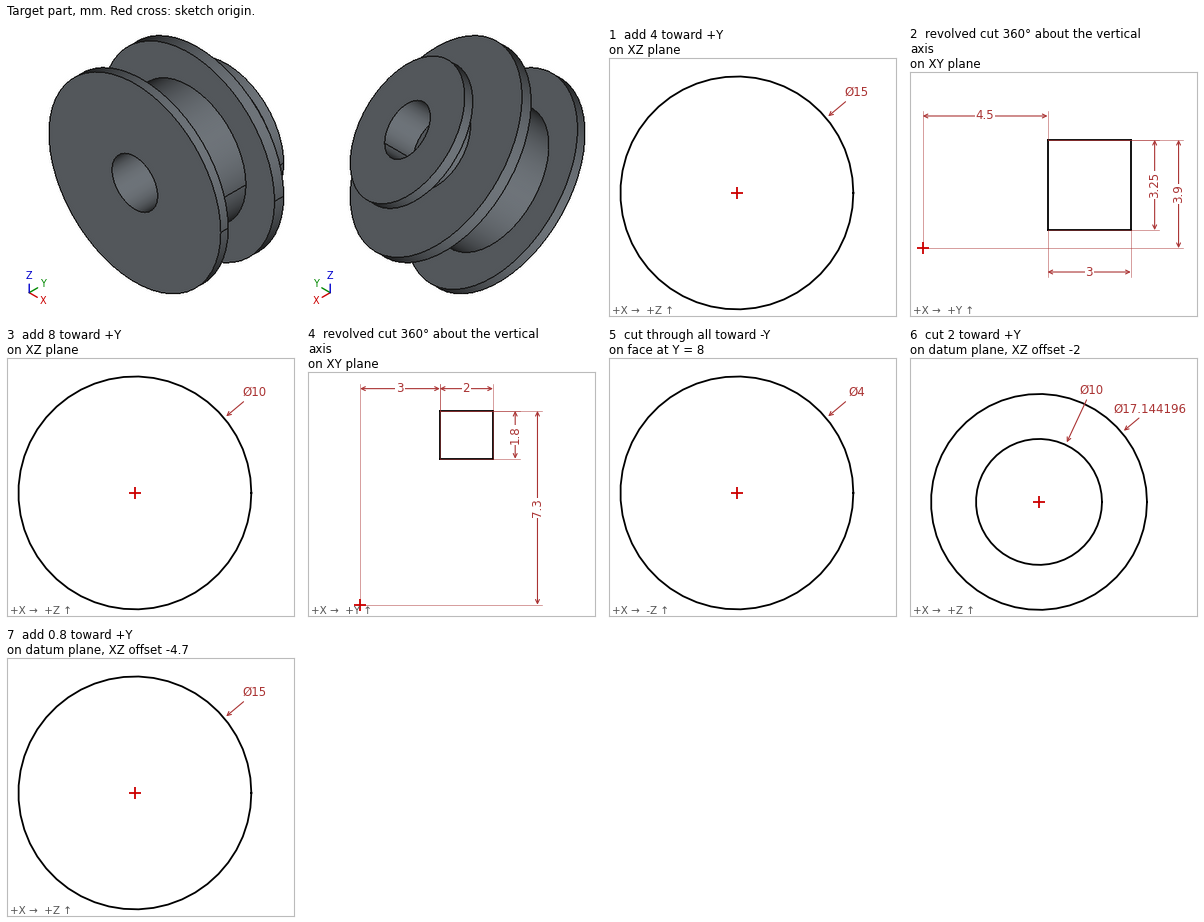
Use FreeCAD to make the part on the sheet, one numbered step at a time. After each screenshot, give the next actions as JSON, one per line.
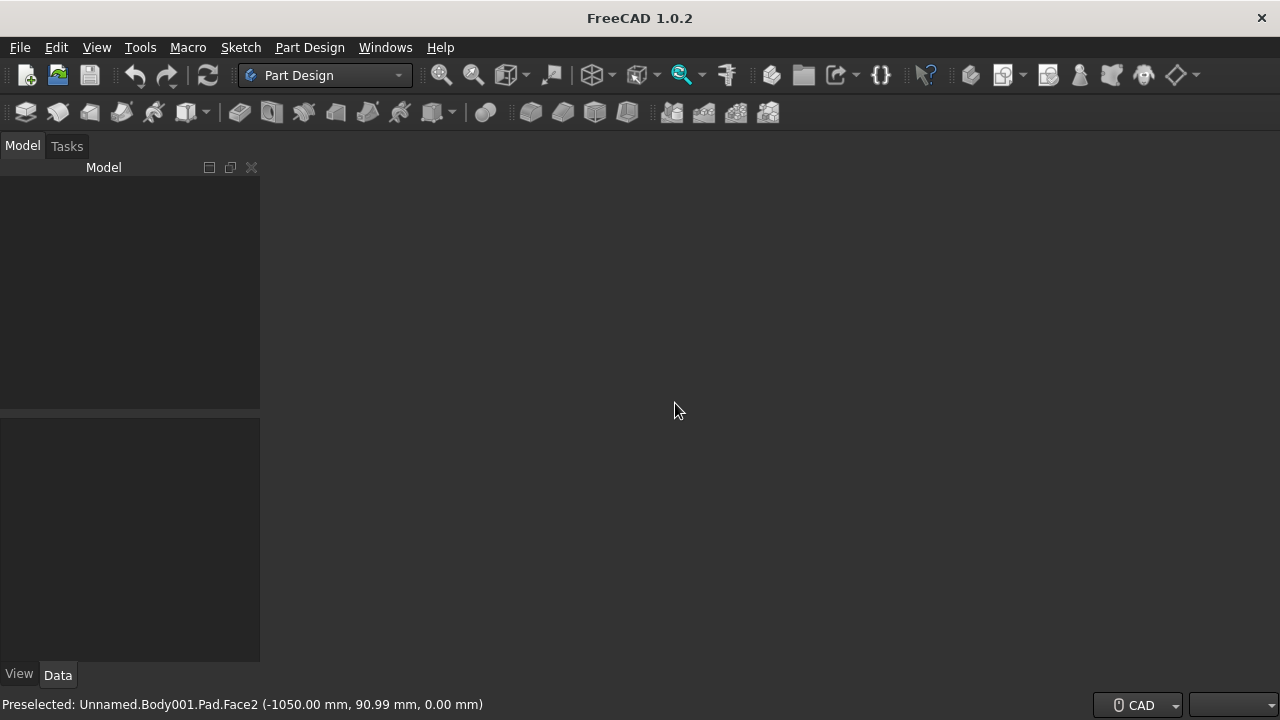
{"action": "left_click", "coordinate": [26, 76]}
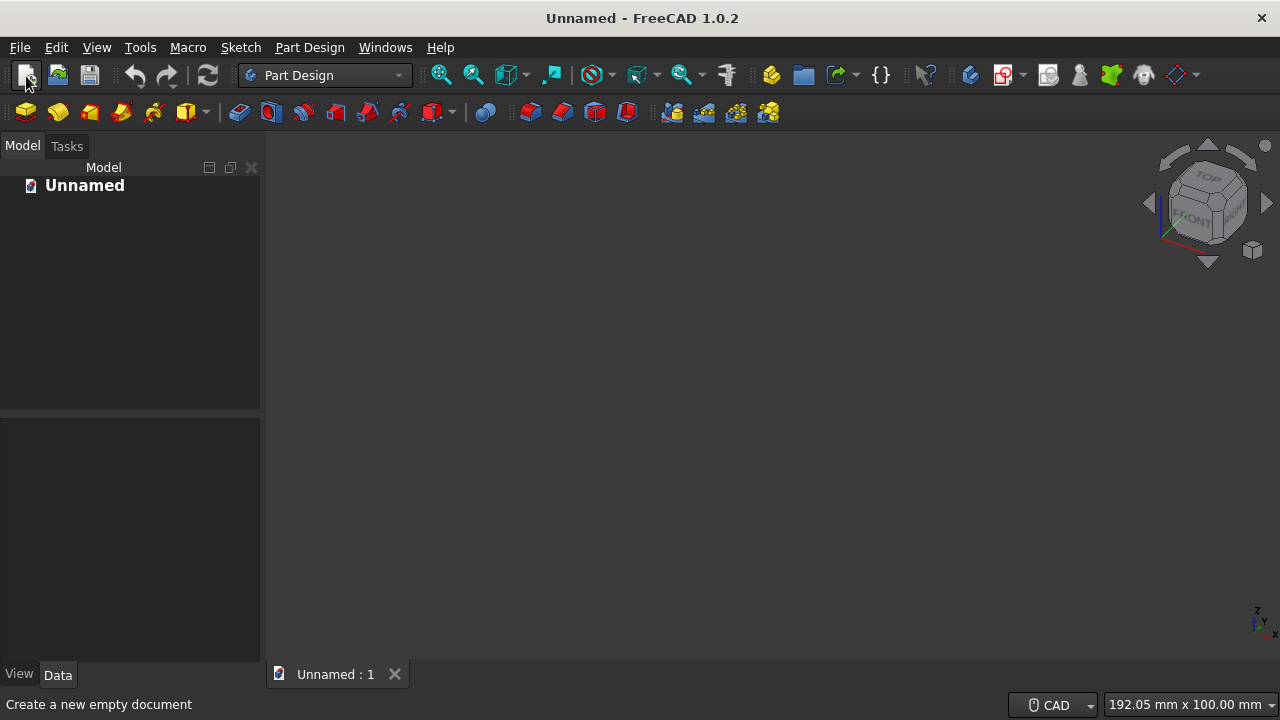
{"action": "left_click", "coordinate": [1004, 76]}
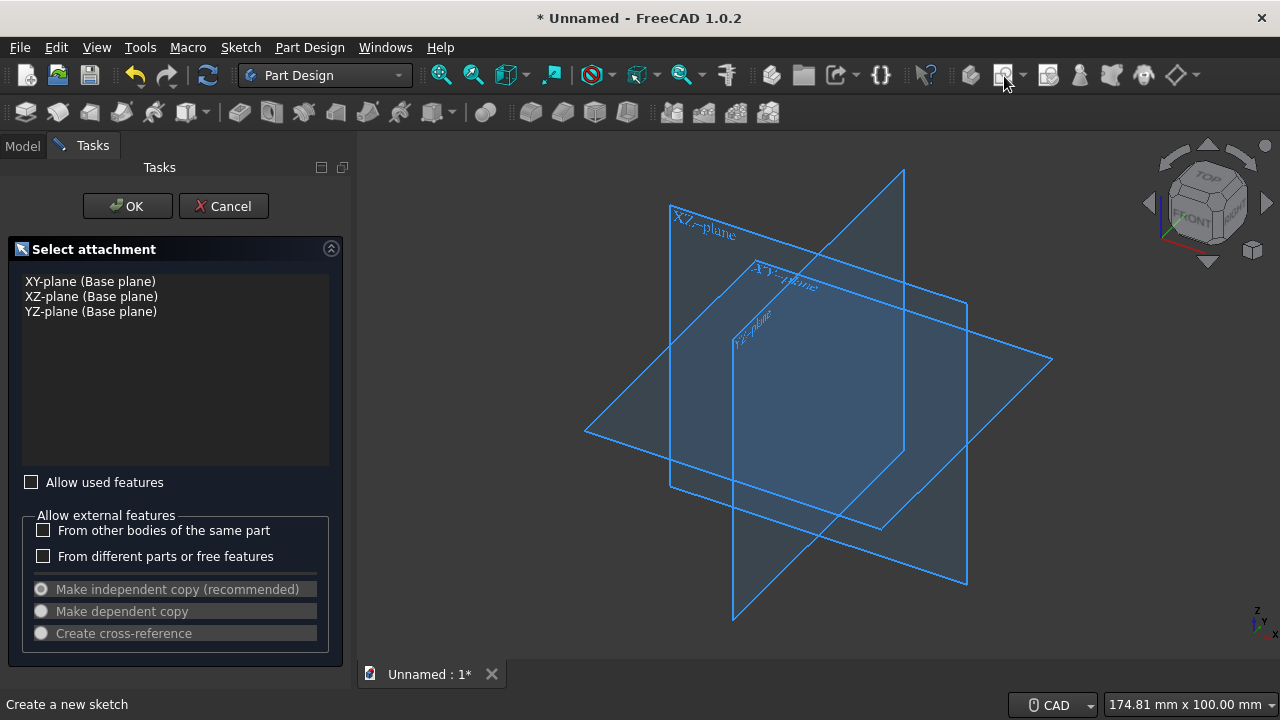
{"action": "left_click", "coordinate": [82, 296]}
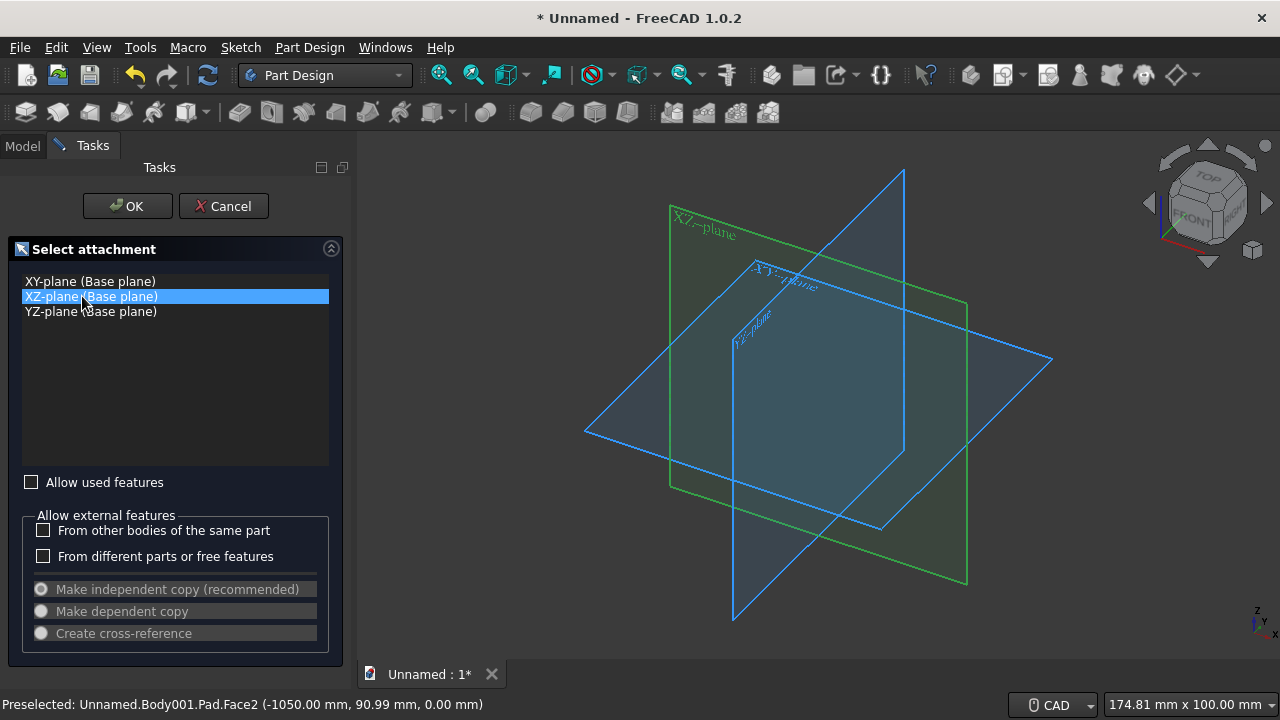
{"action": "left_click", "coordinate": [128, 206]}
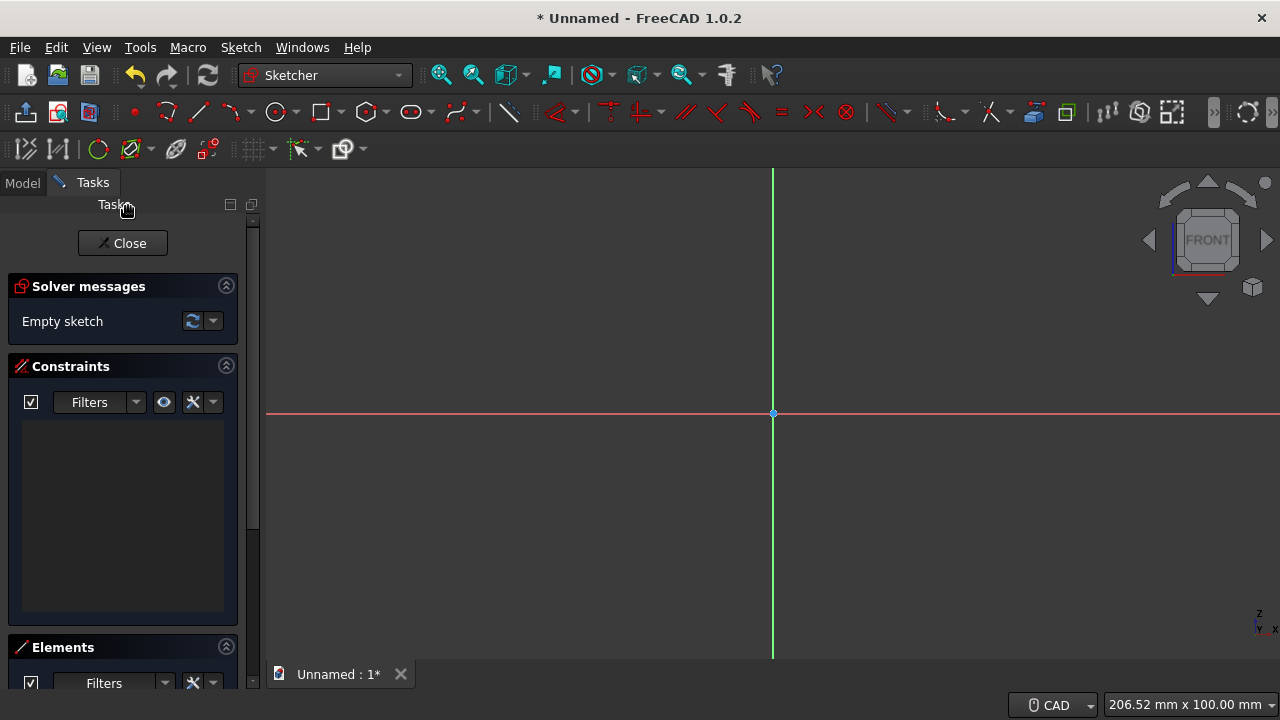
{"action": "scroll", "coordinate": [795, 414], "scroll_direction": "up", "scroll_amount": 7}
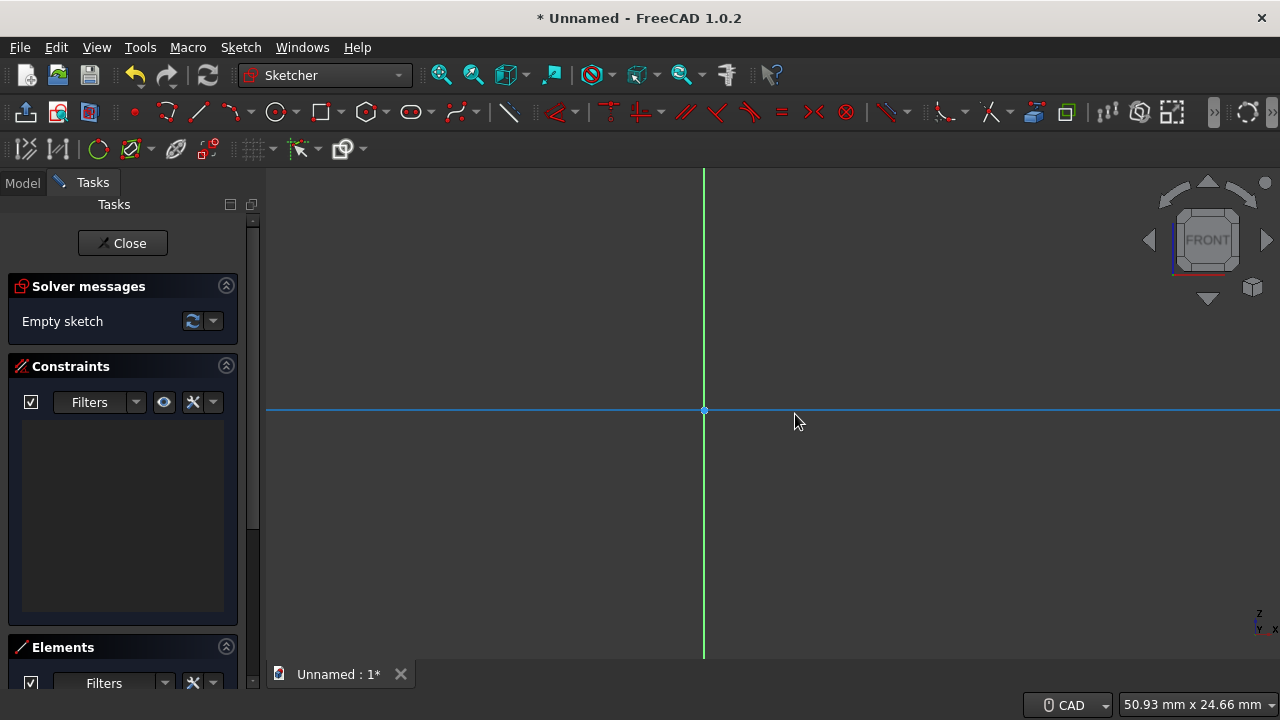
{"action": "left_click", "coordinate": [276, 112]}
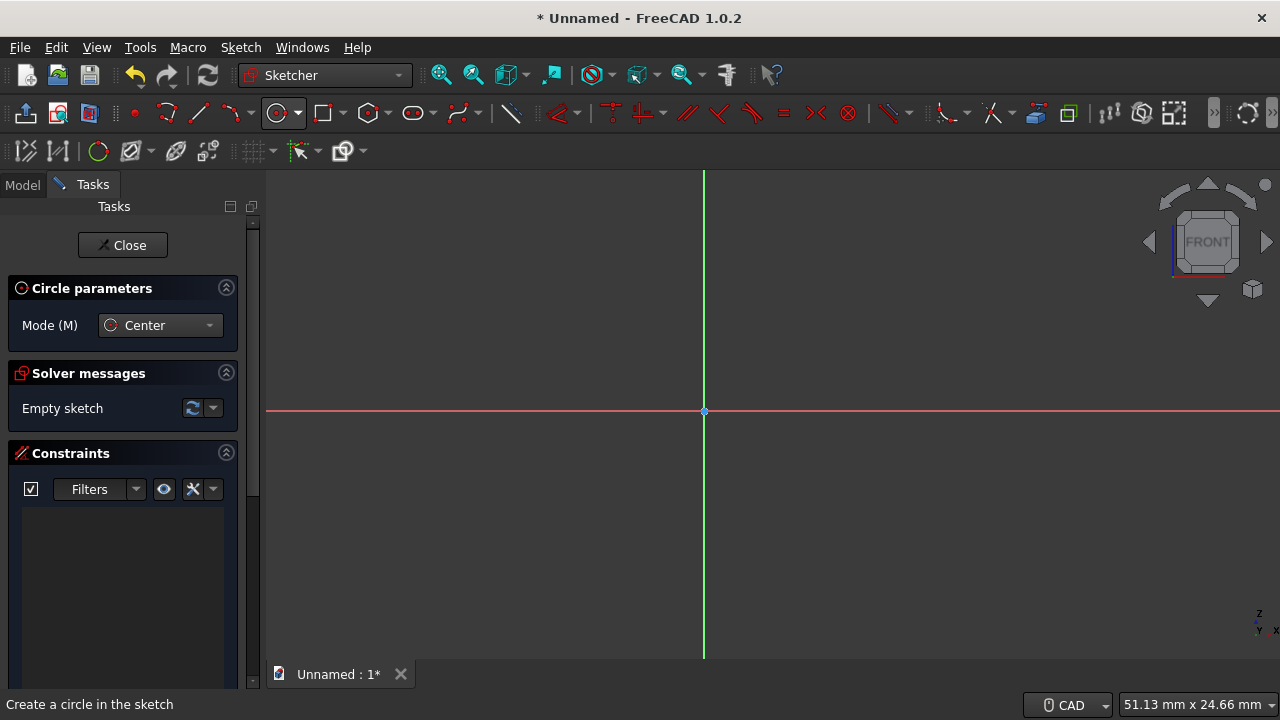
{"action": "left_click", "coordinate": [704, 411]}
{"action": "left_click", "coordinate": [810, 306]}
{"action": "key", "text": "Escape"}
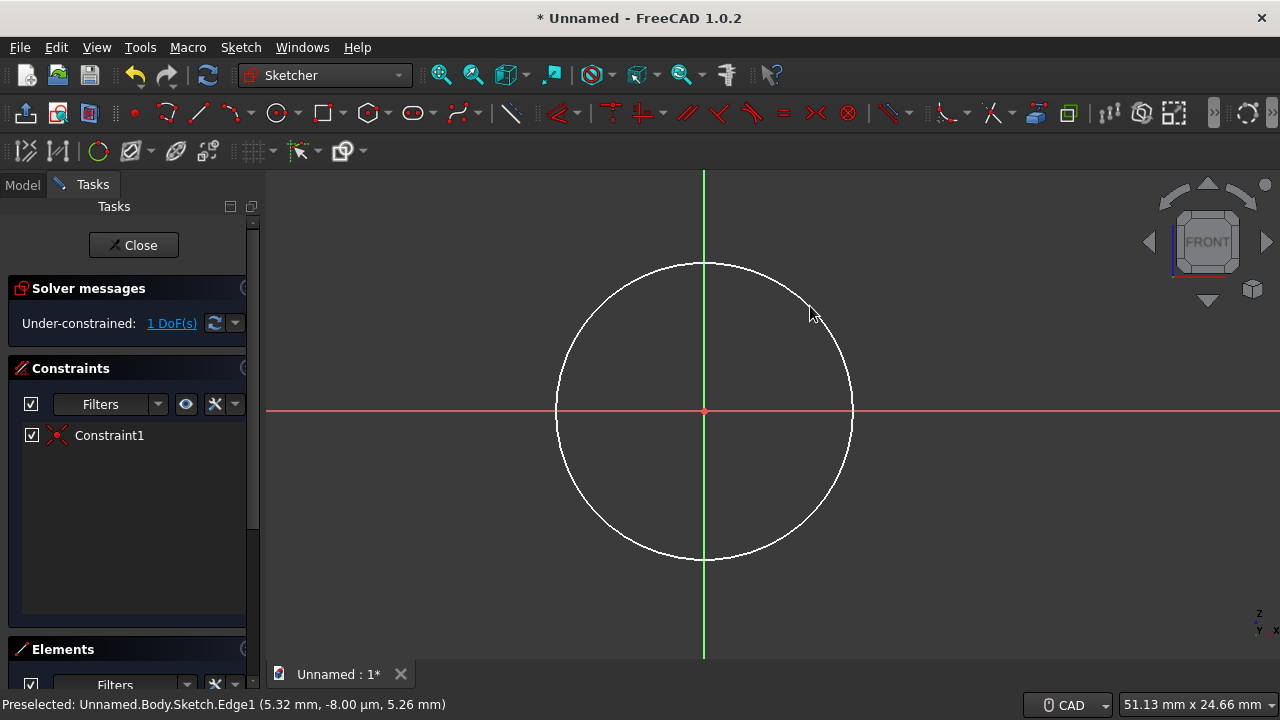
{"action": "left_click", "coordinate": [558, 114]}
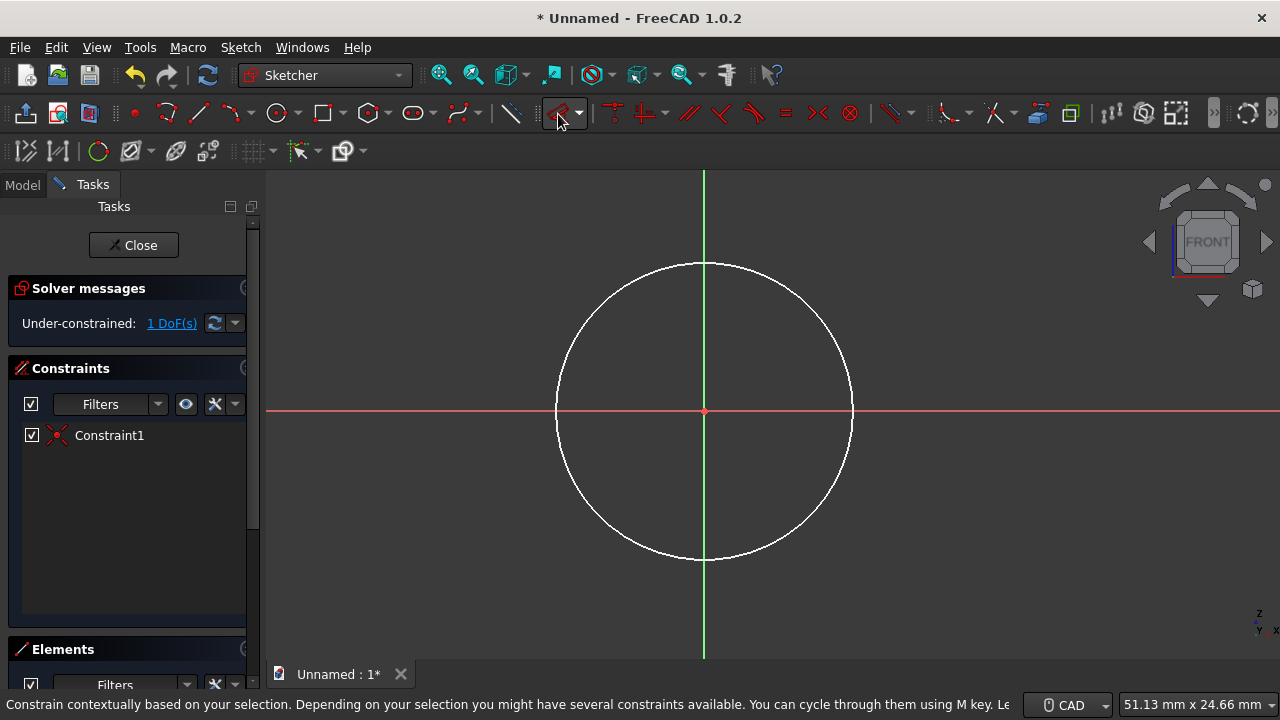
{"action": "left_click", "coordinate": [809, 306]}
{"action": "left_click", "coordinate": [832, 283]}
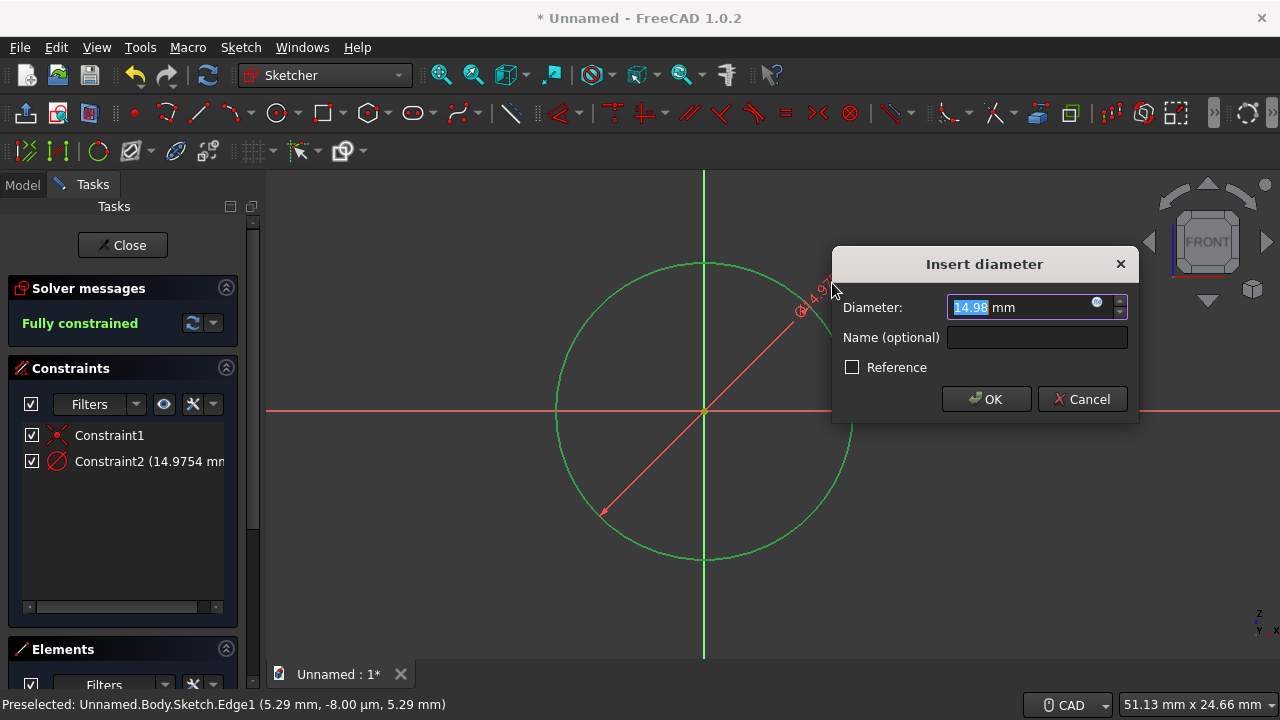
{"action": "type", "text": "15"}
{"action": "key", "text": "Return"}
{"action": "key", "text": "Escape"}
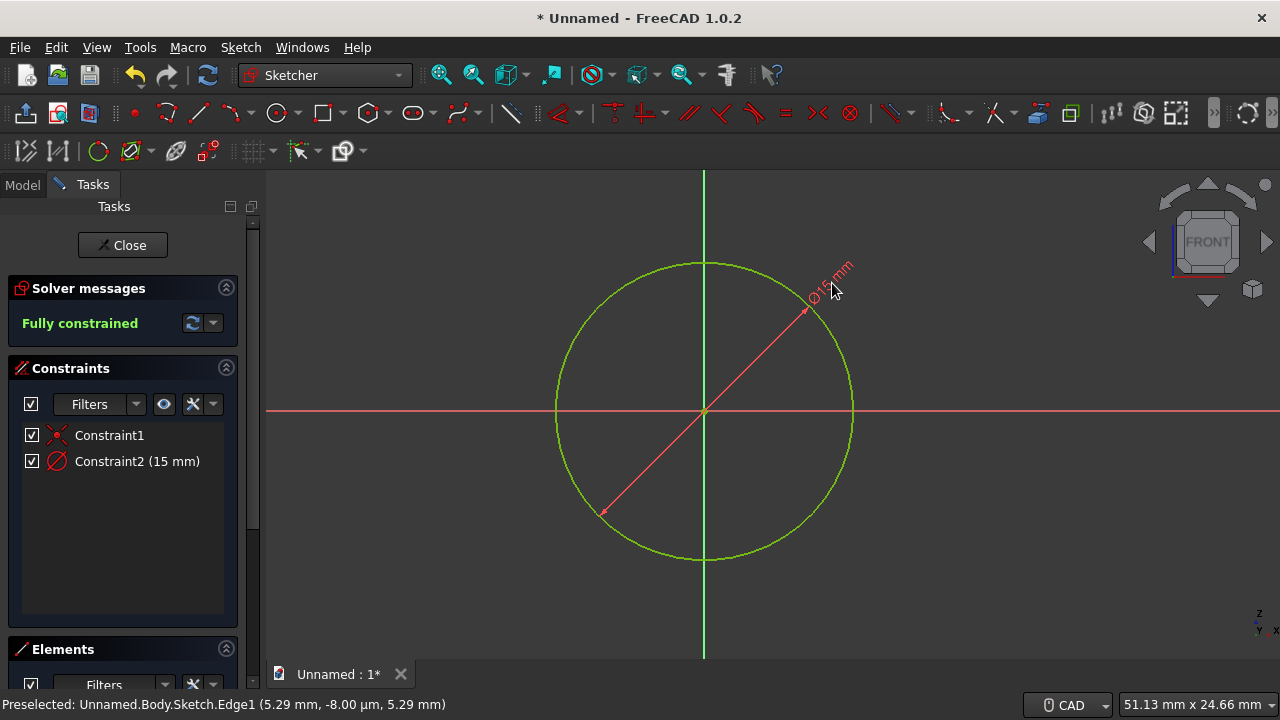
{"action": "left_click", "coordinate": [123, 245]}